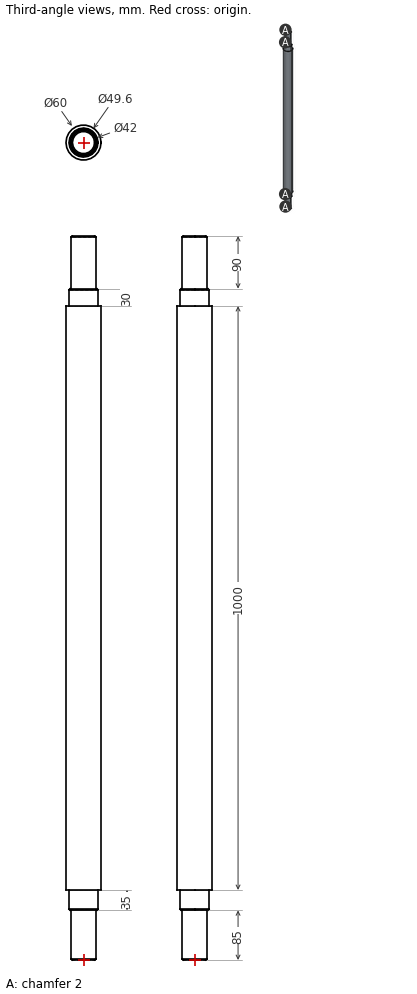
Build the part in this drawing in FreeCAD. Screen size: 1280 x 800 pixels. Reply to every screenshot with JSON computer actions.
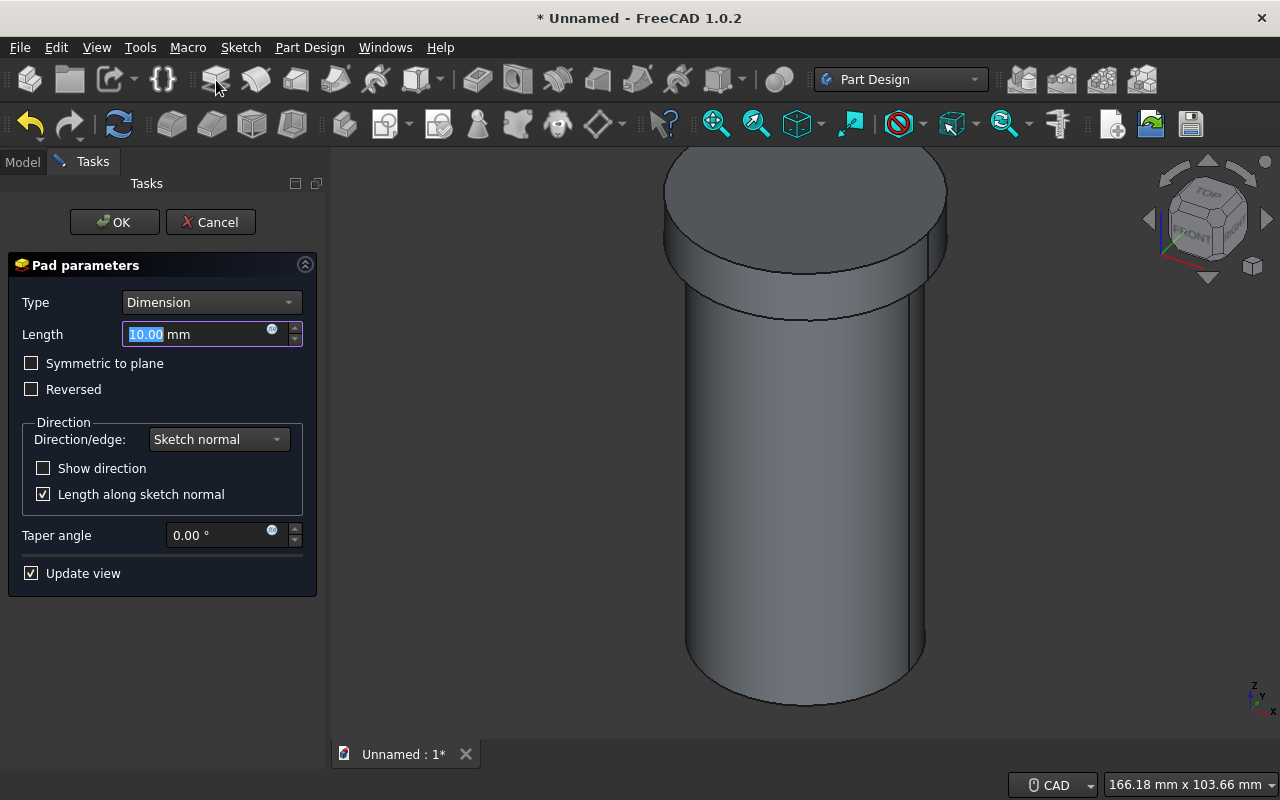
{"action": "type", "text": "35"}
{"action": "key", "text": "Tab"}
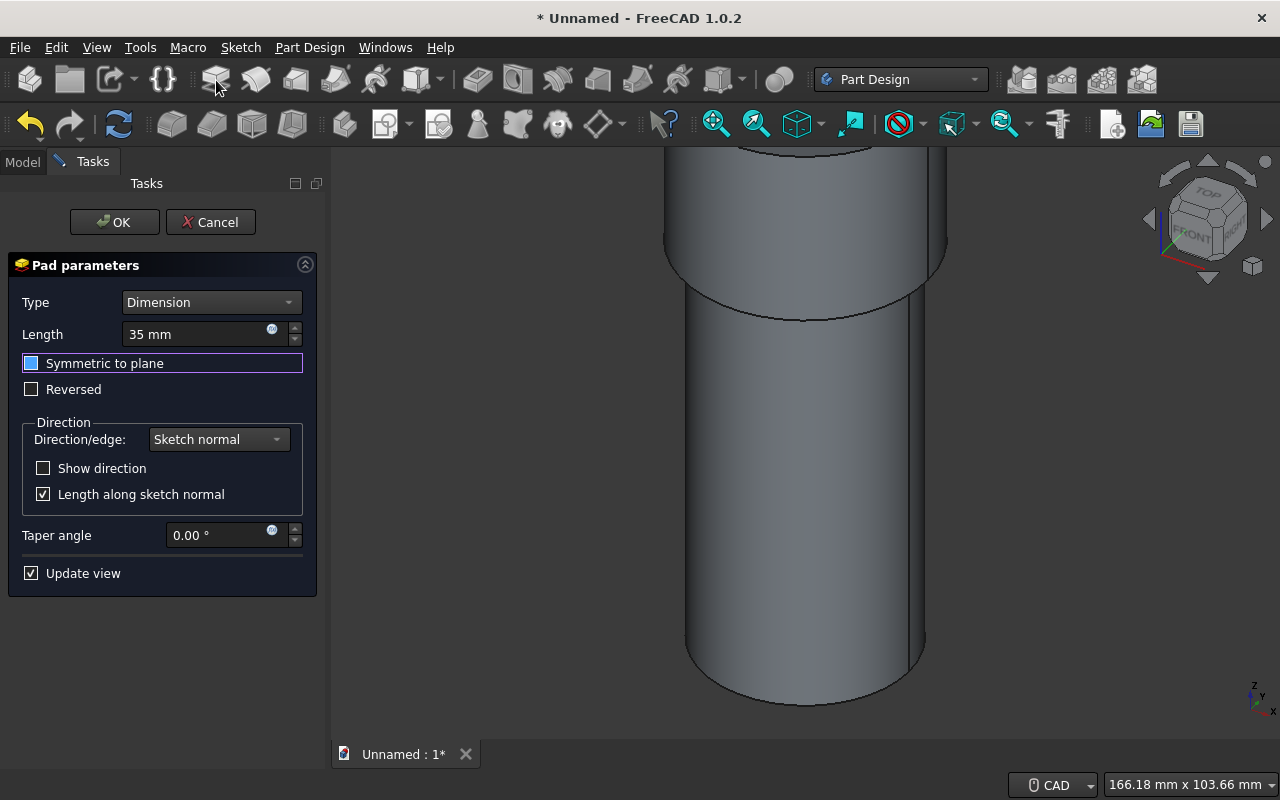
{"action": "left_click", "coordinate": [115, 222]}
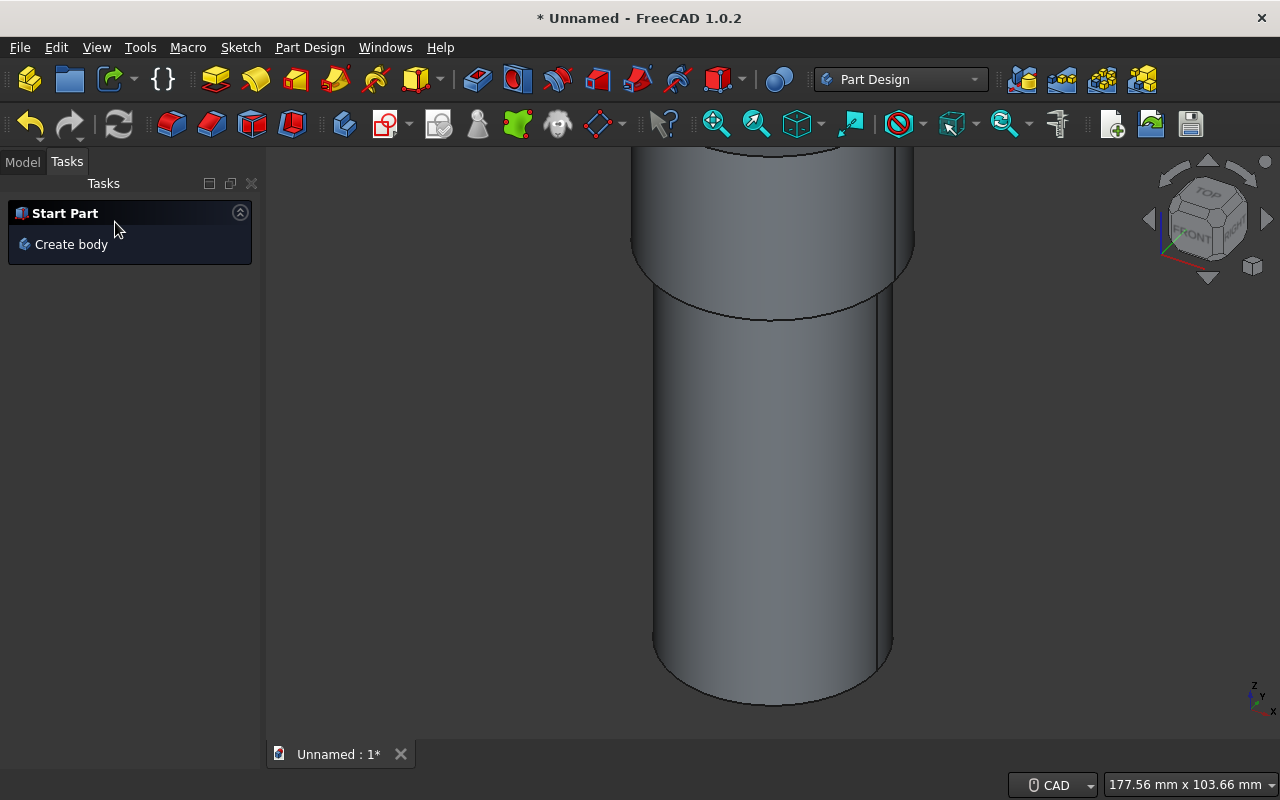
{"action": "key", "text": "v f"}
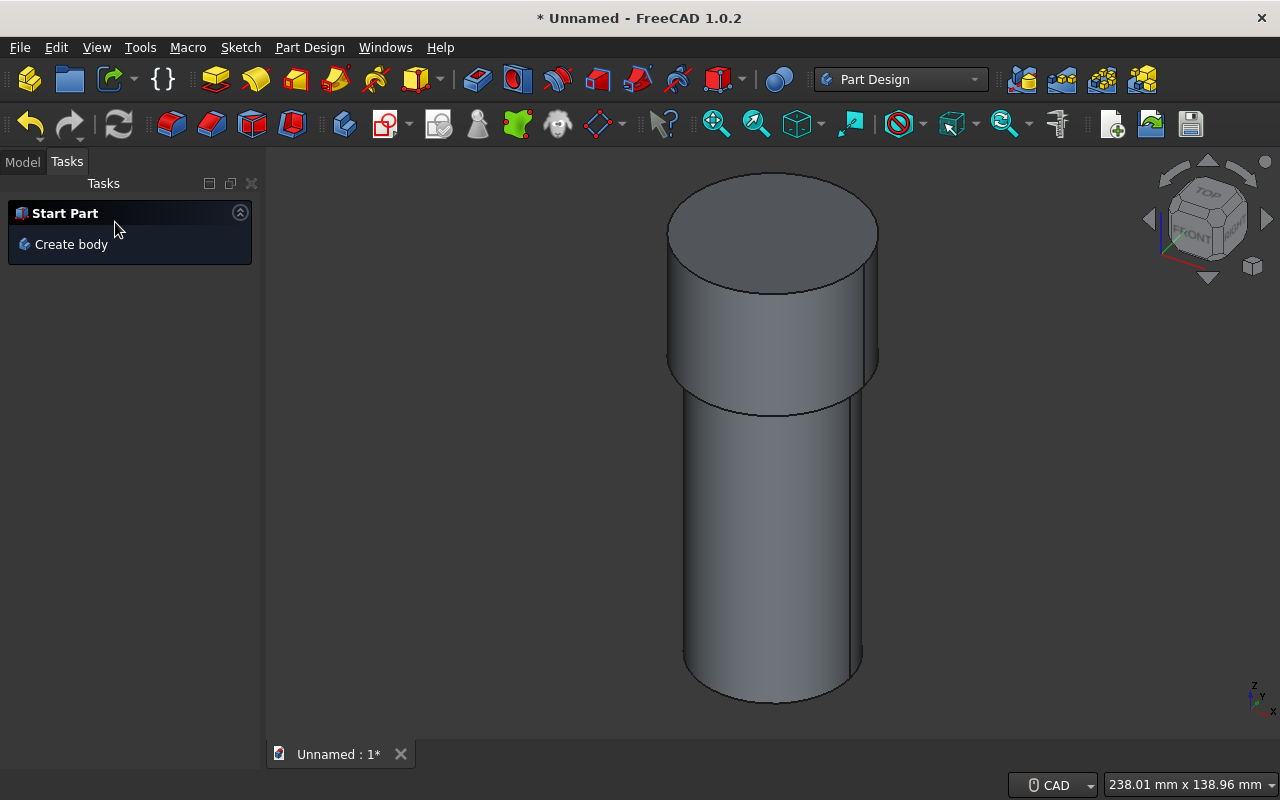
{"action": "left_click", "coordinate": [773, 233]}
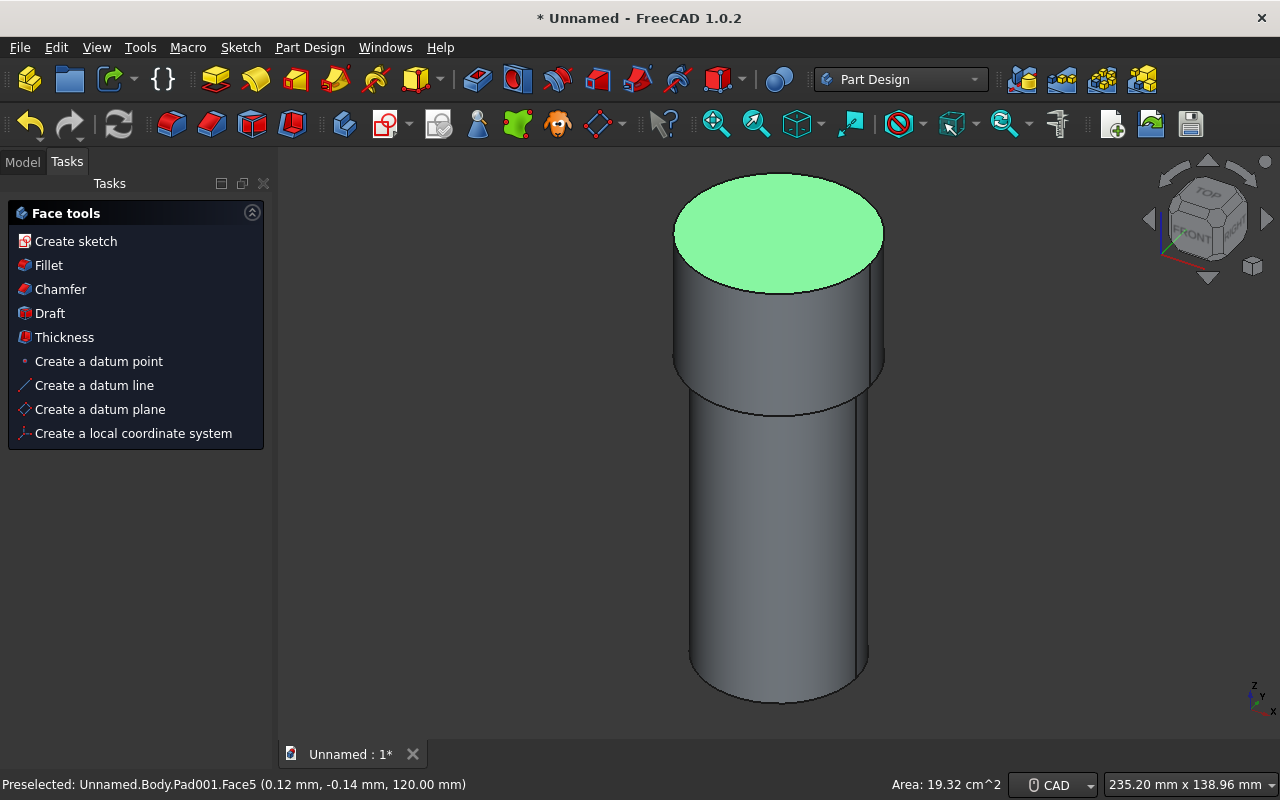
{"action": "left_click", "coordinate": [386, 124]}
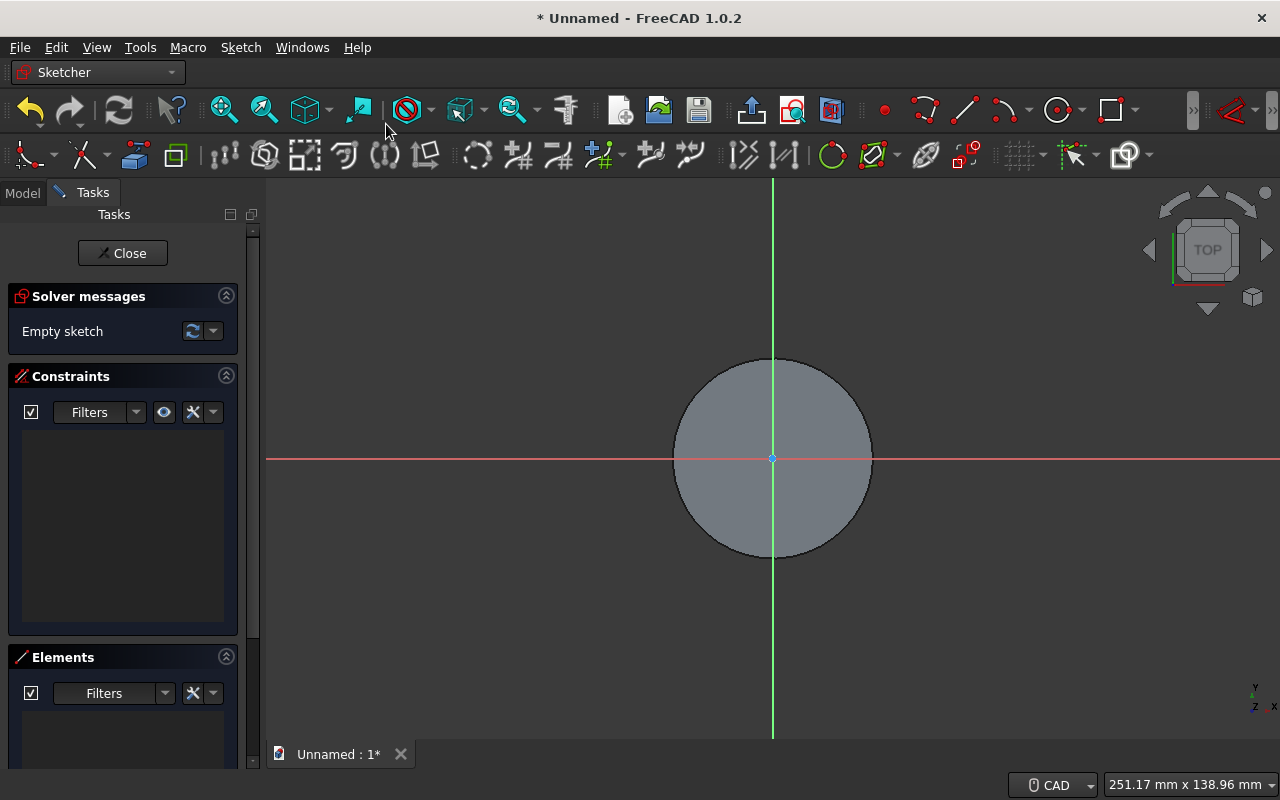
{"action": "scroll", "coordinate": [912, 458], "scroll_direction": "up", "scroll_amount": 2}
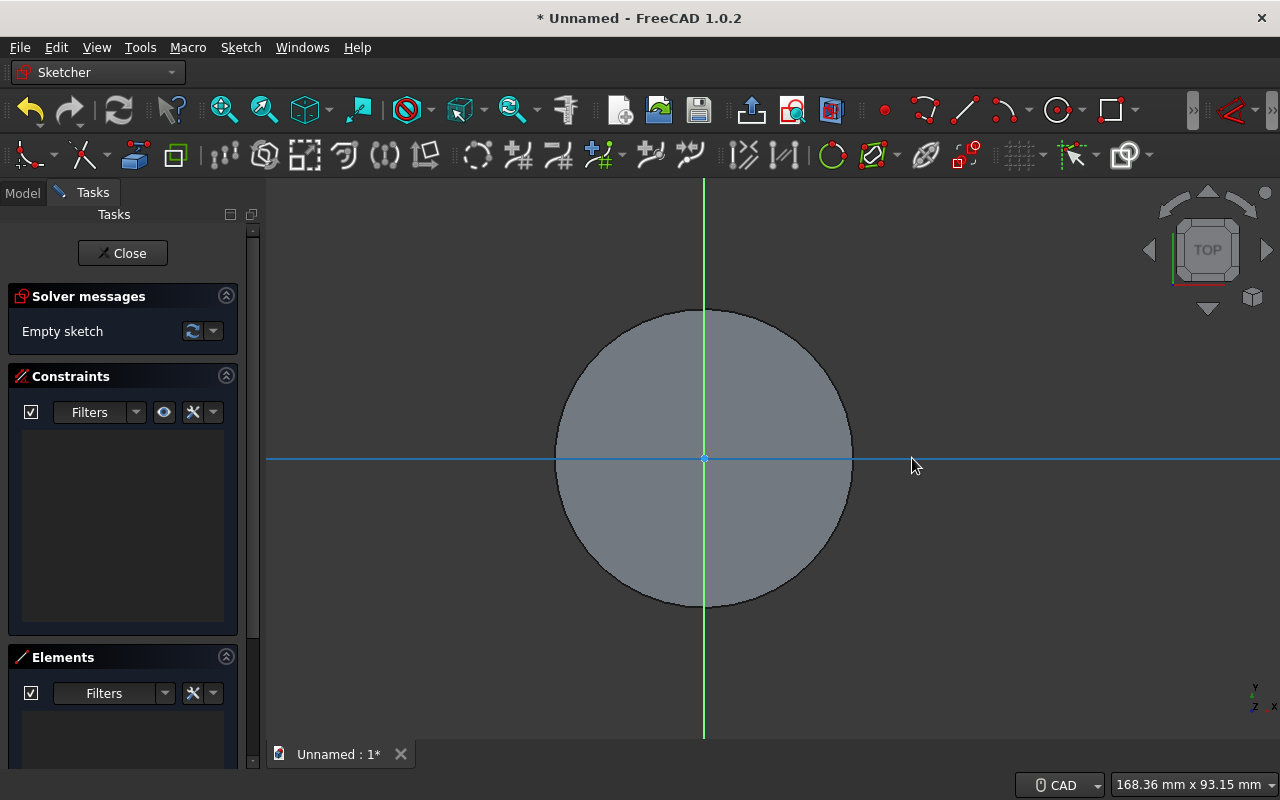
{"action": "key", "text": "g c"}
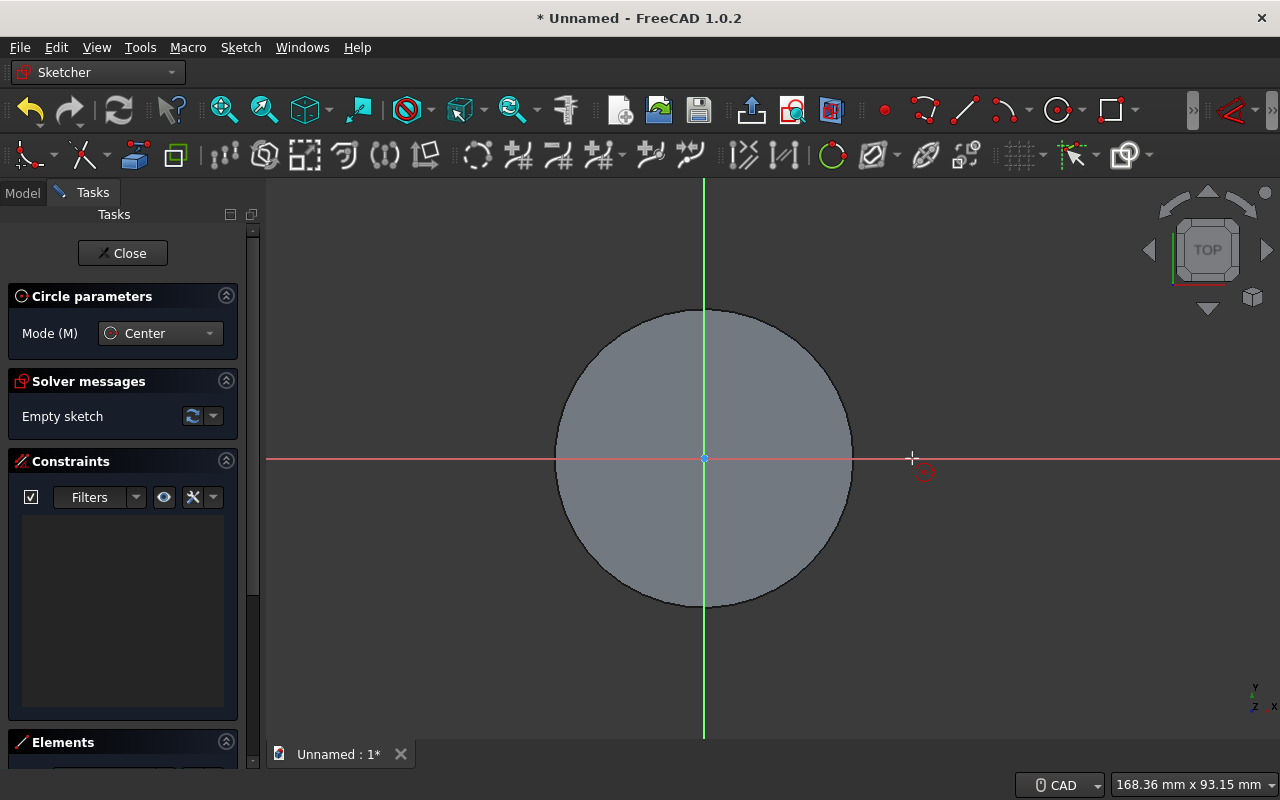
{"action": "left_click", "coordinate": [704, 458]}
{"action": "mouse_move", "coordinate": [832, 331]}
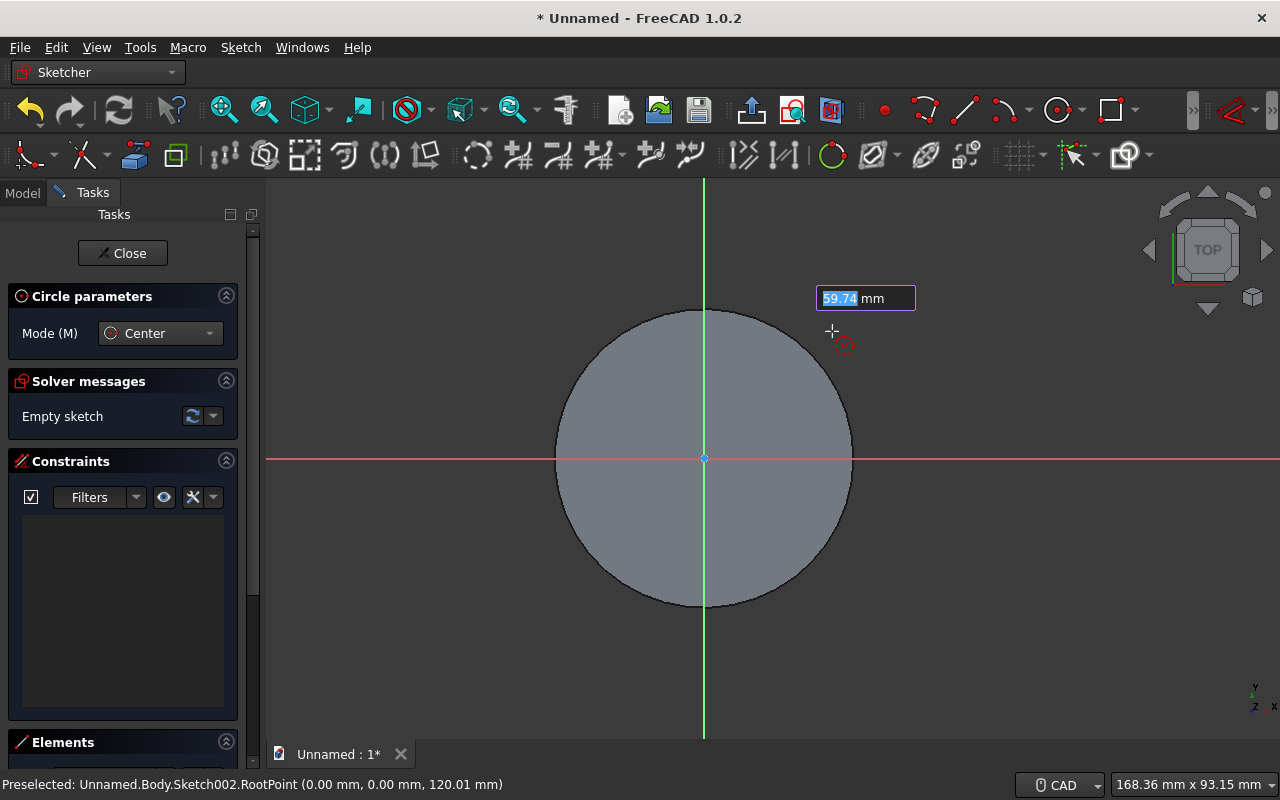
{"action": "type", "text": "60"}
{"action": "key", "text": "Return"}
{"action": "key", "text": "Escape"}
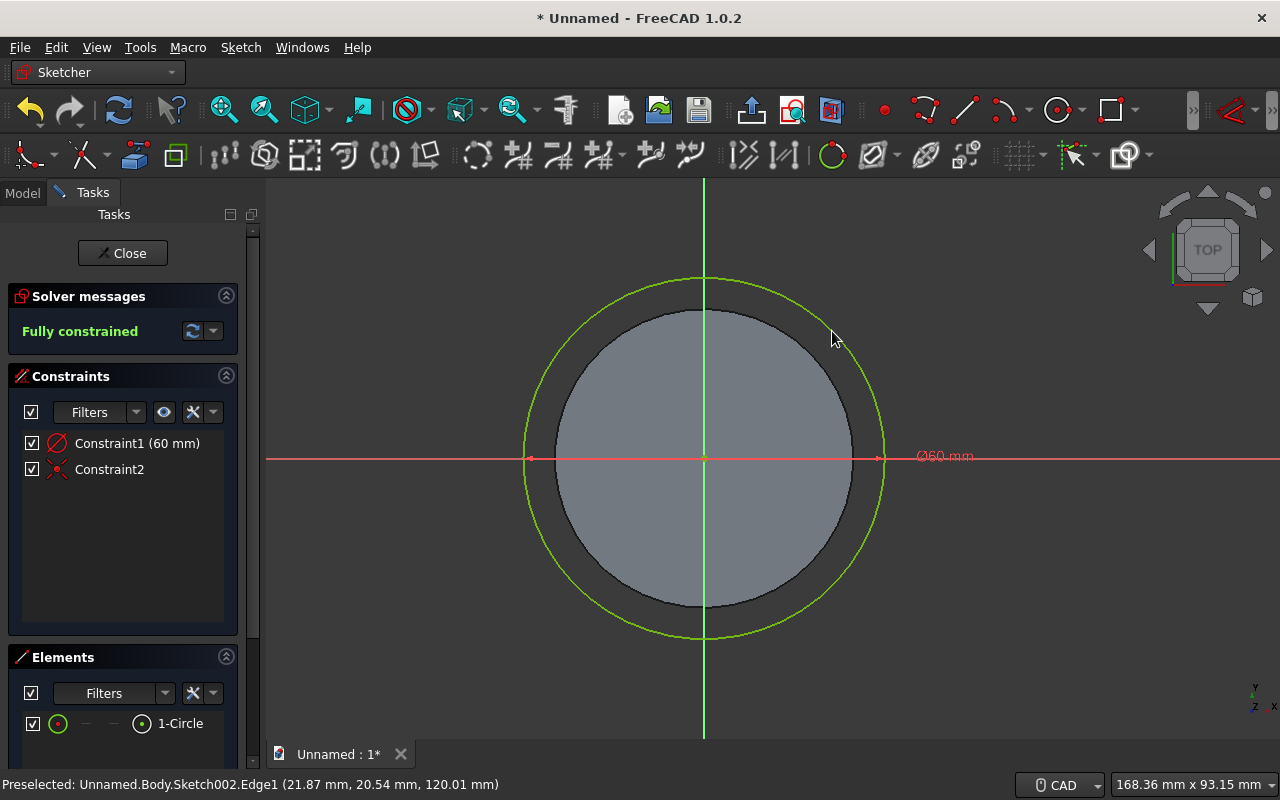
{"action": "left_click", "coordinate": [123, 253]}